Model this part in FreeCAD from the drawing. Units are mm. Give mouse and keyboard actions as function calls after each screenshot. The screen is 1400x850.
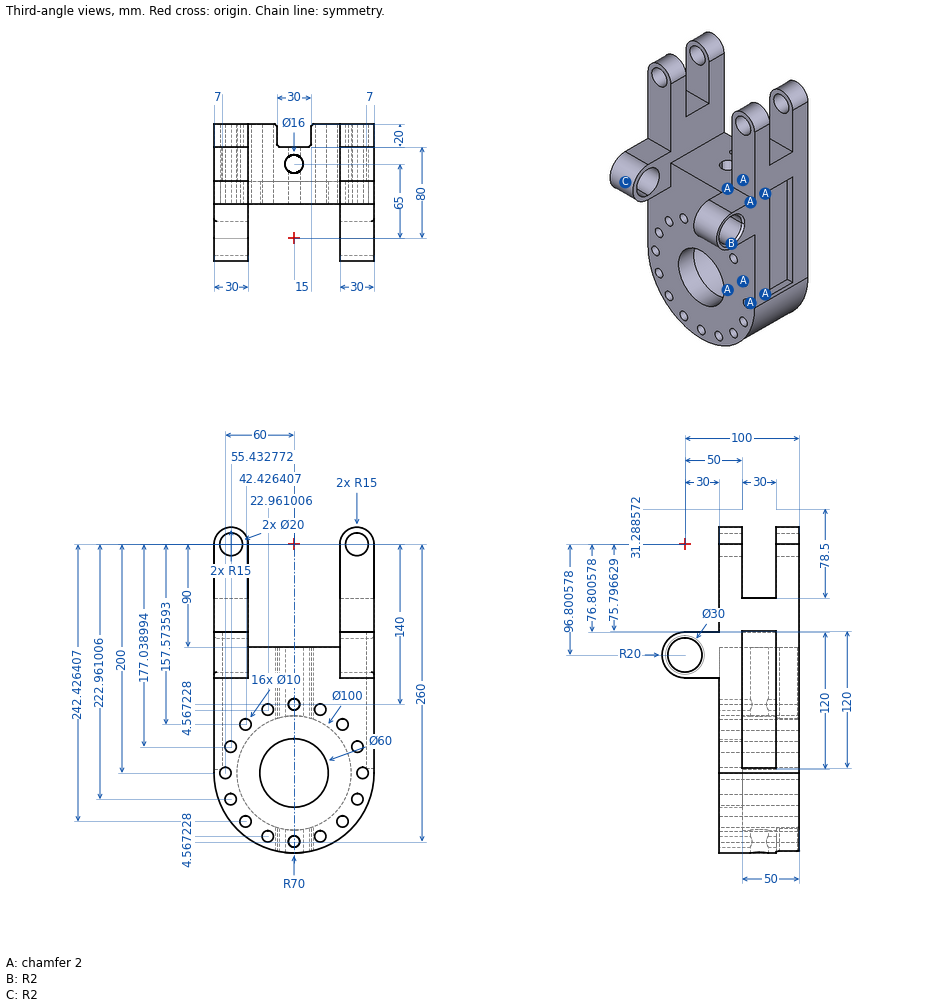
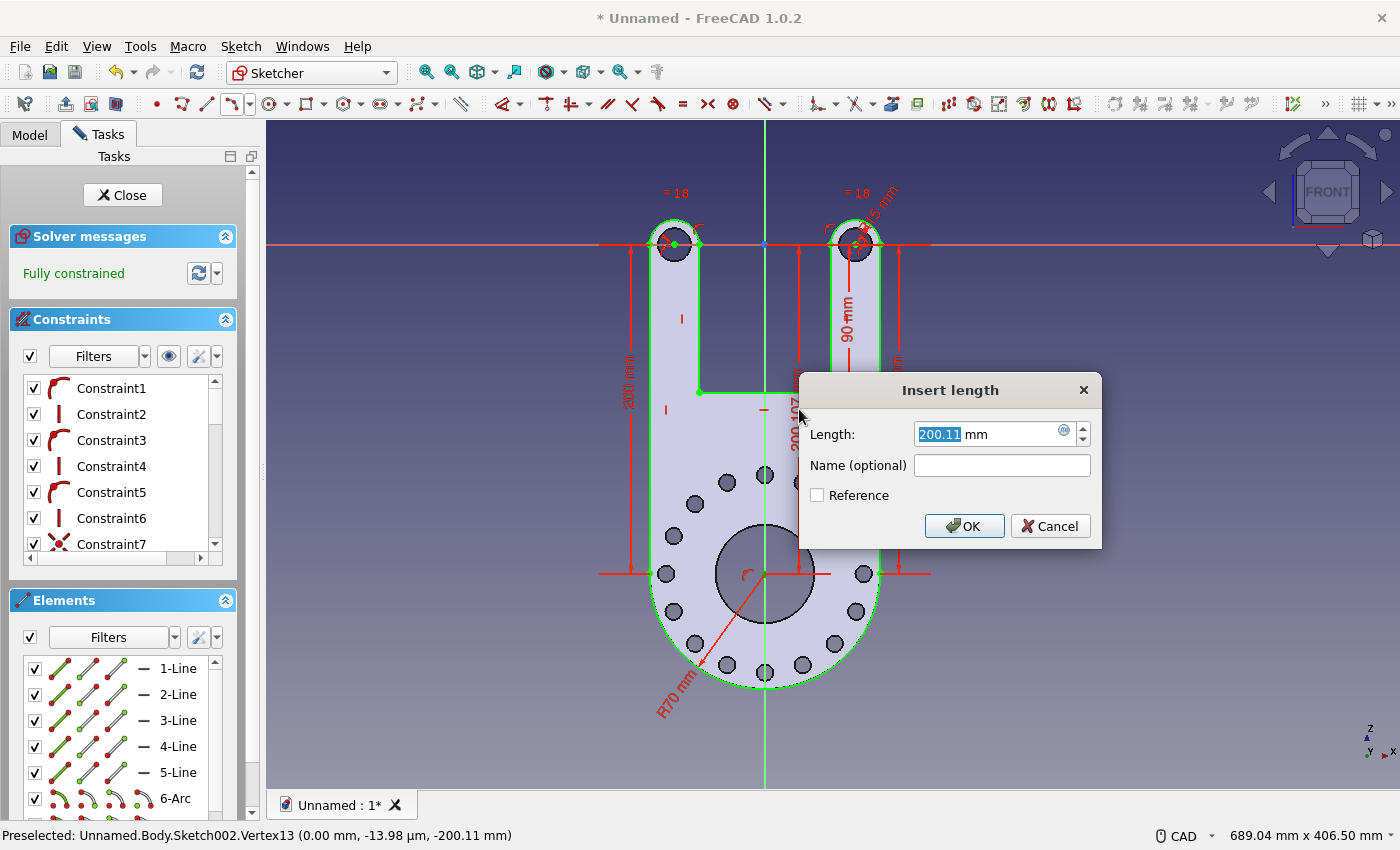
text(200)
key(Return)
key(Escape)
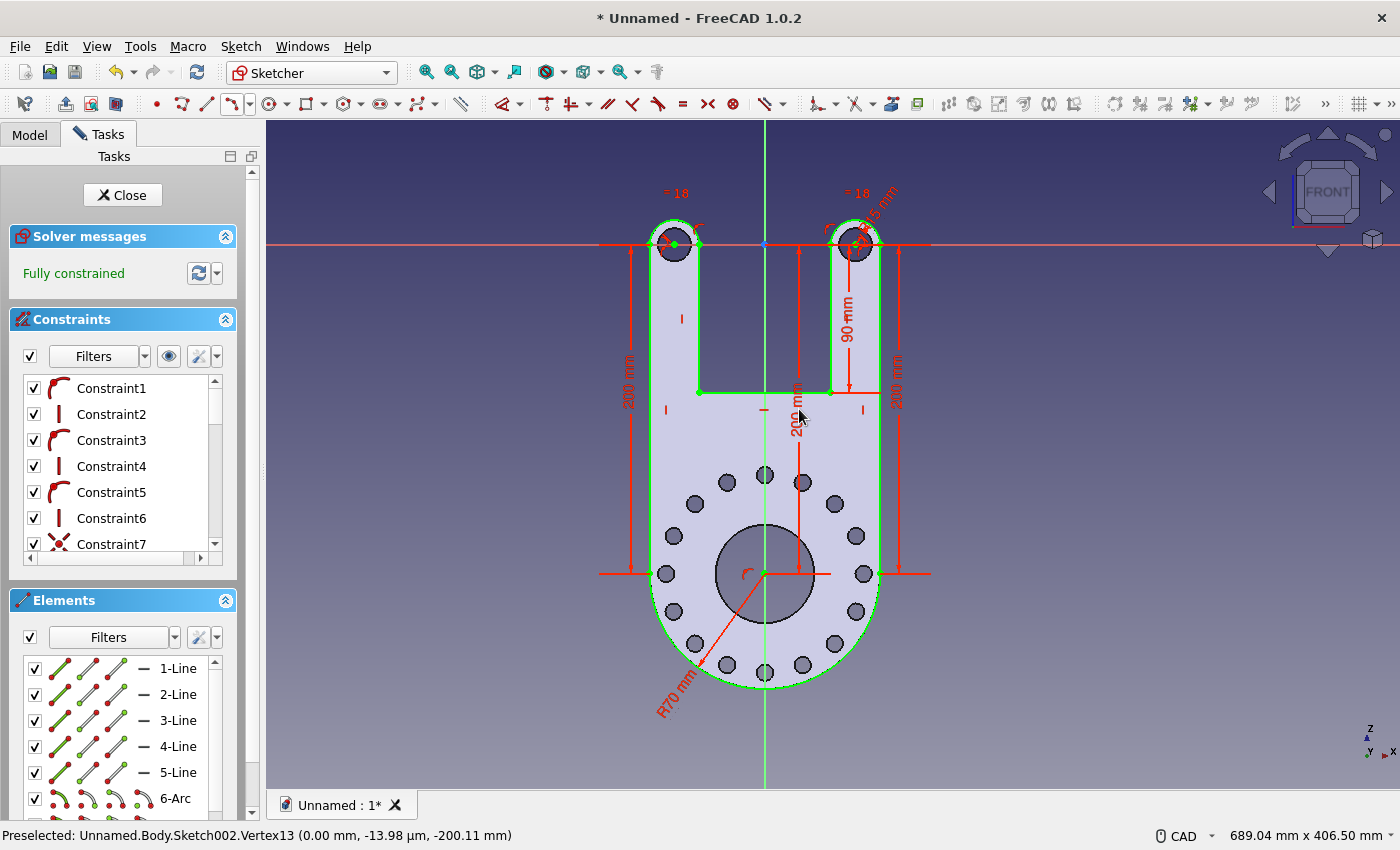
click(123, 195)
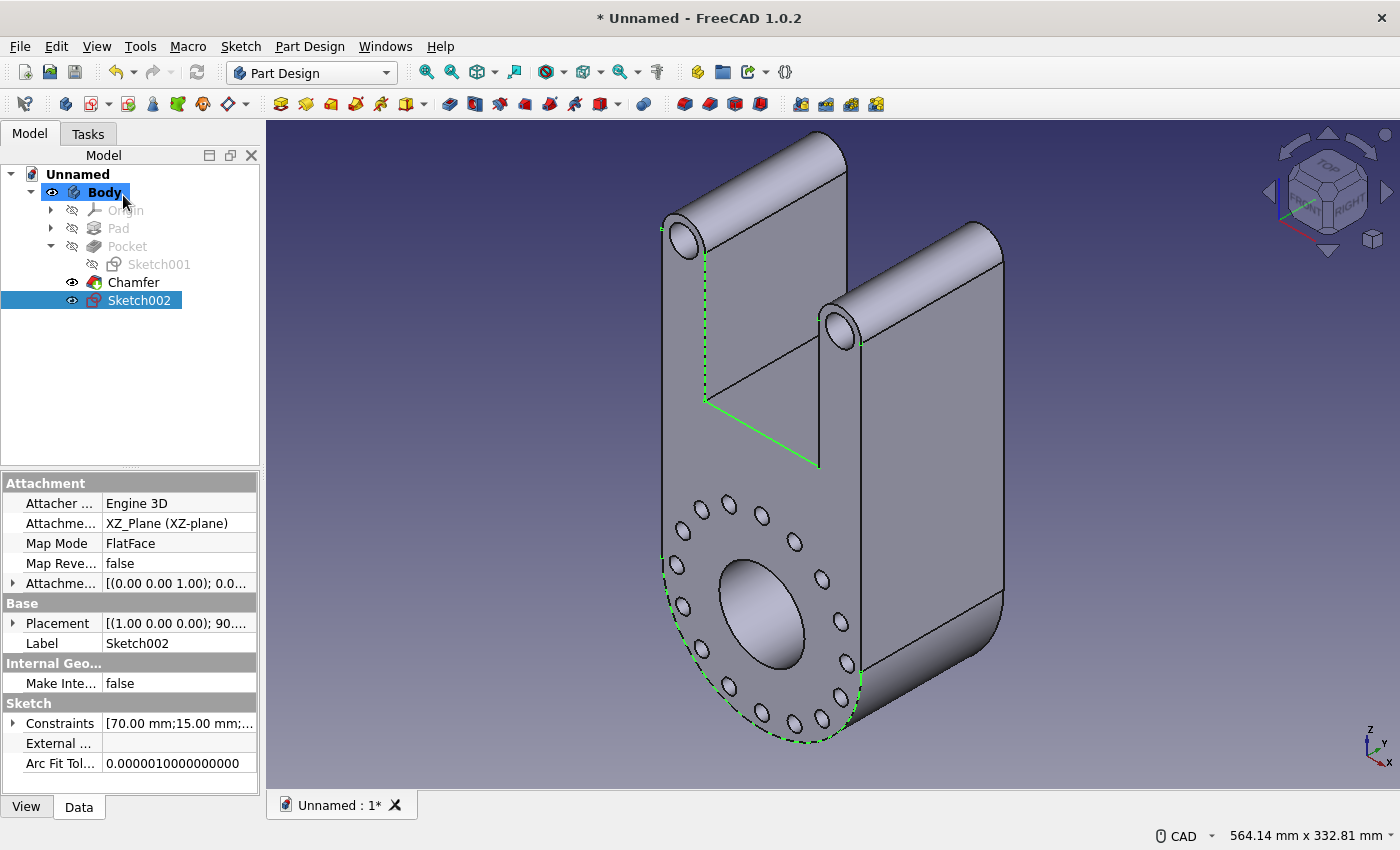
click(450, 104)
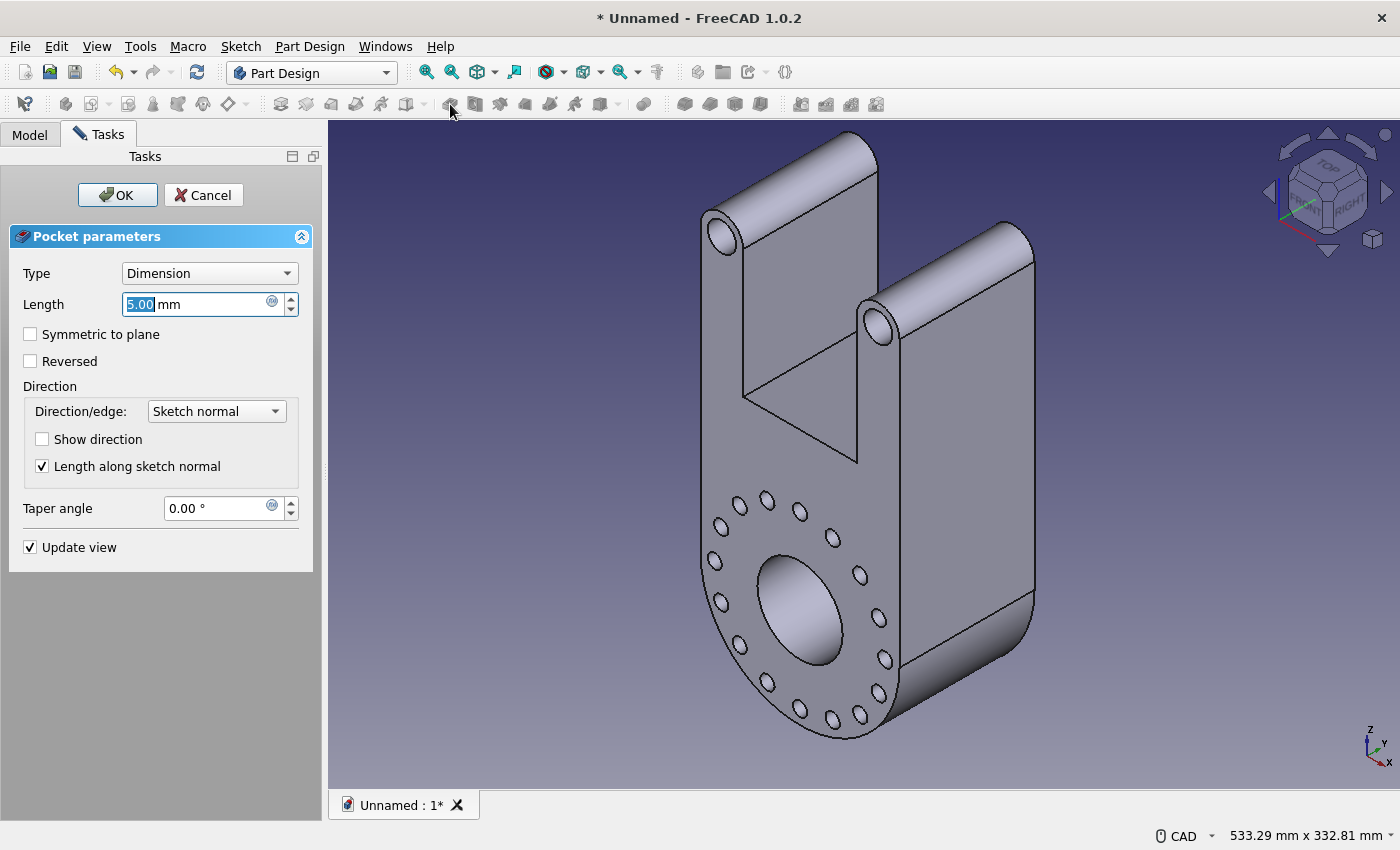
text(30)
key(Tab)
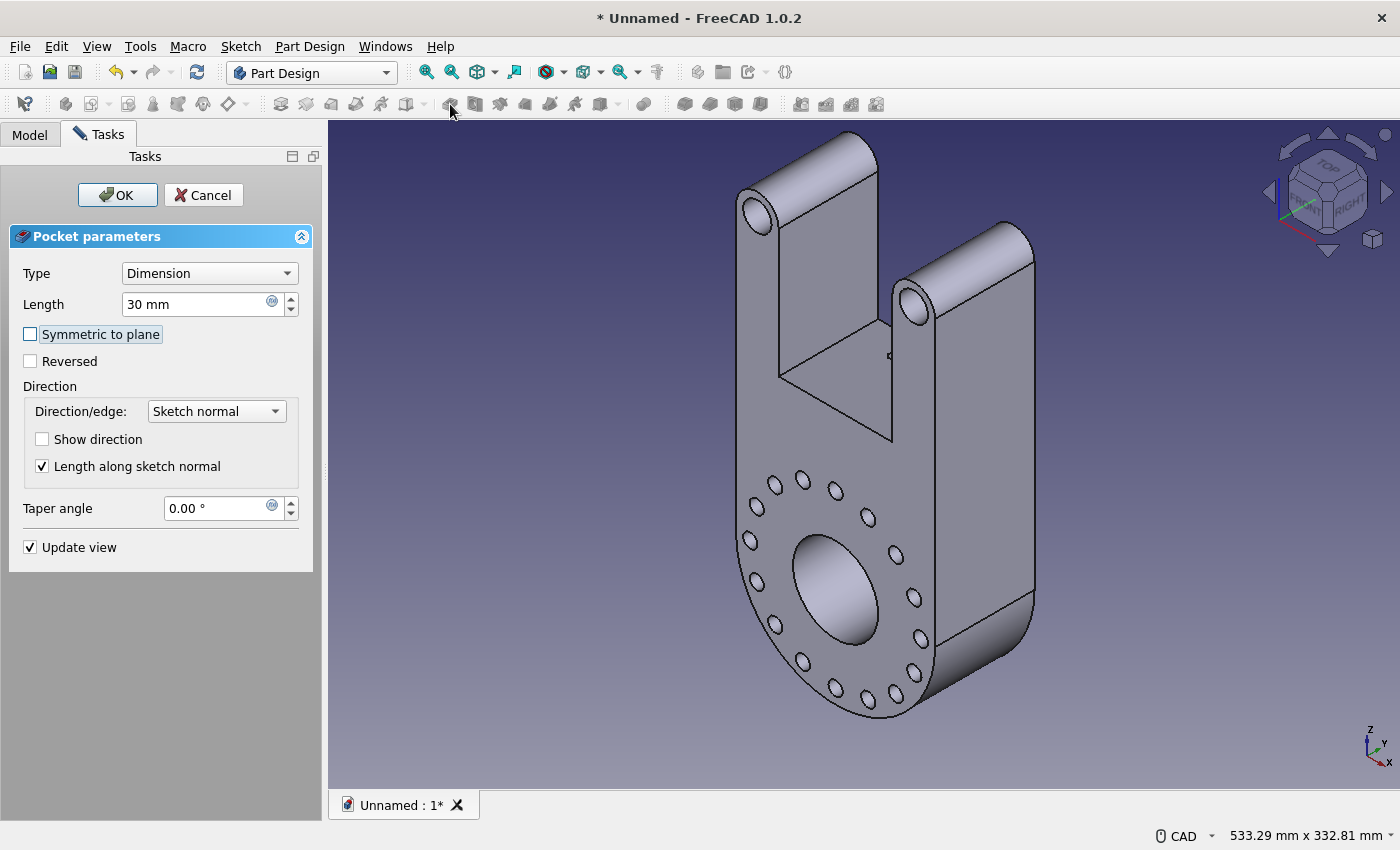
click(118, 195)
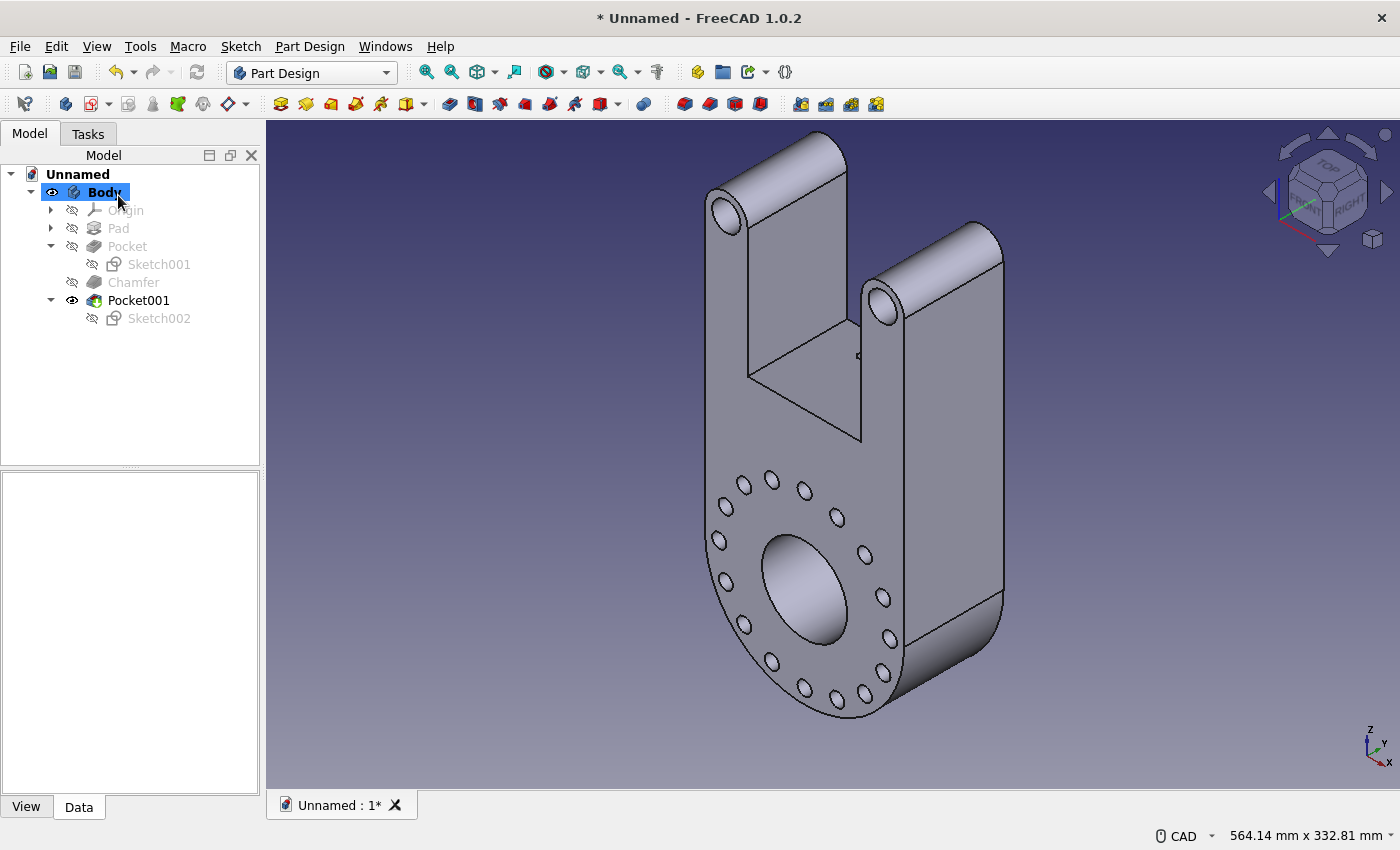
key(4)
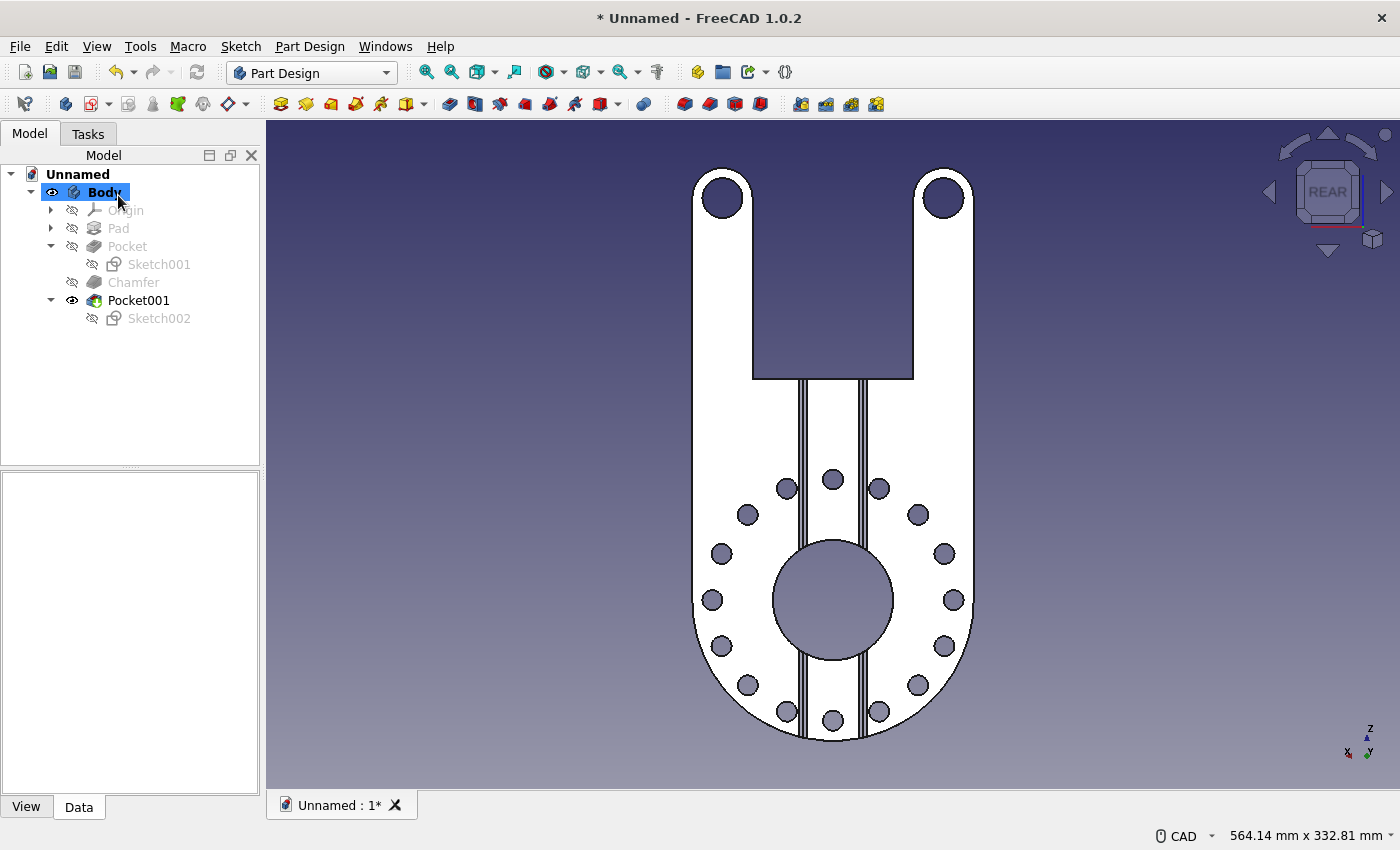
click(920, 451)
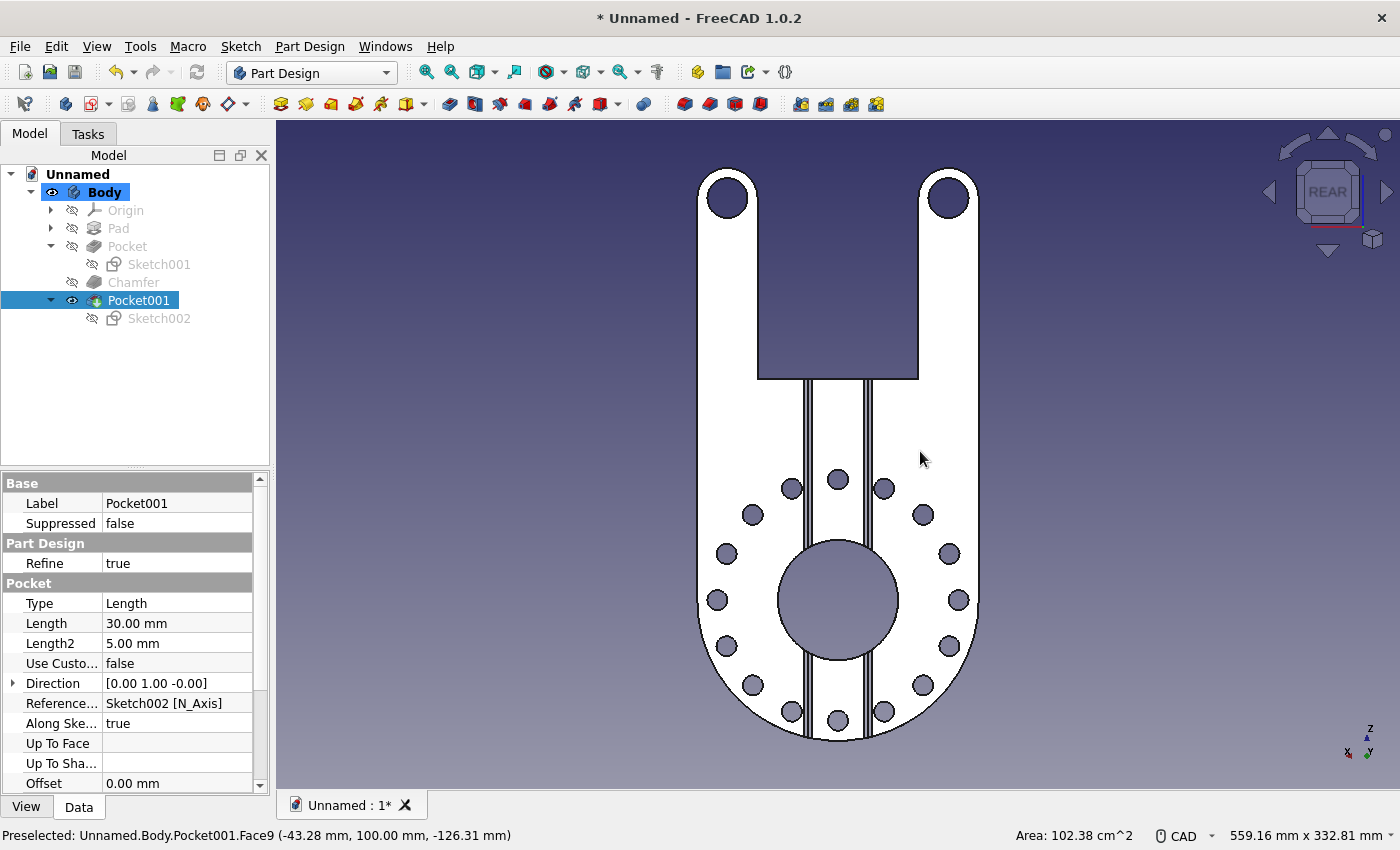
click(90, 104)